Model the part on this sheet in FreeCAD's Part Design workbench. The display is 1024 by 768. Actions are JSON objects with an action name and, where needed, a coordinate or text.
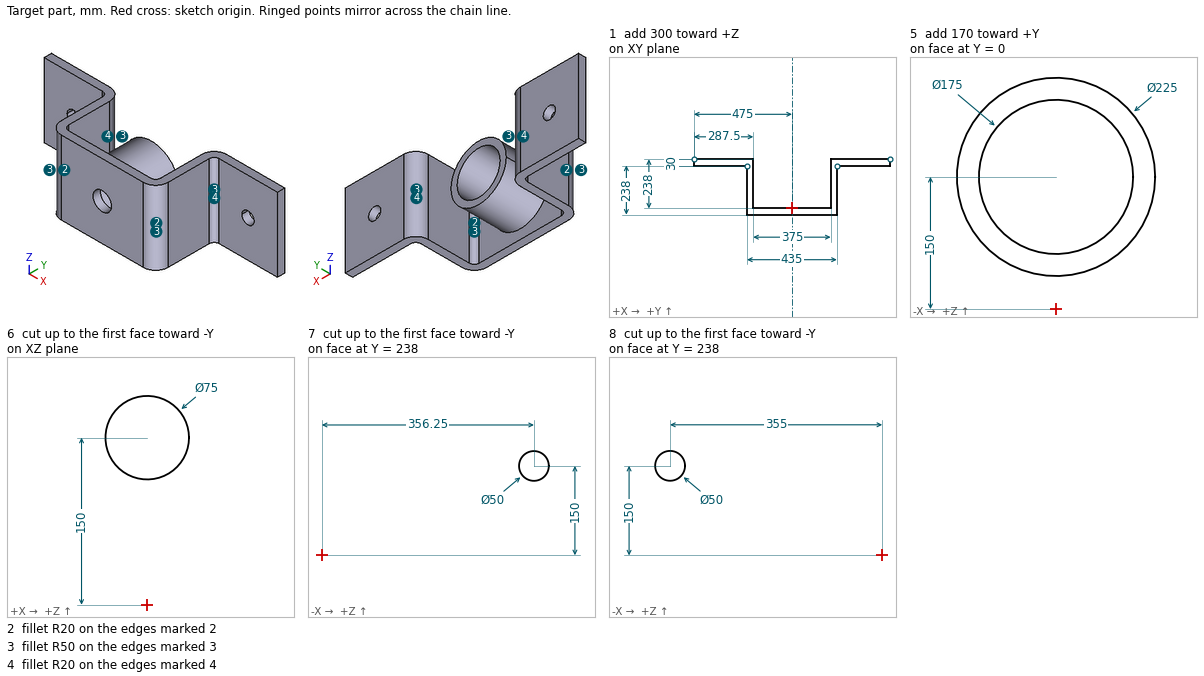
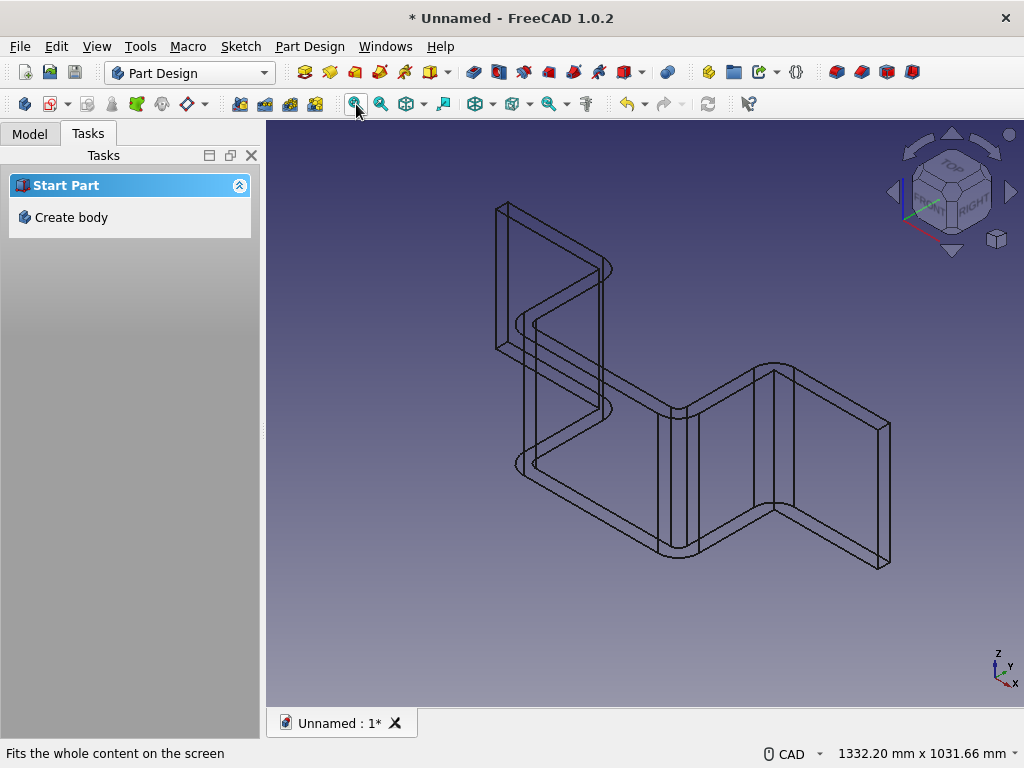
{"action": "left_click", "coordinate": [774, 439]}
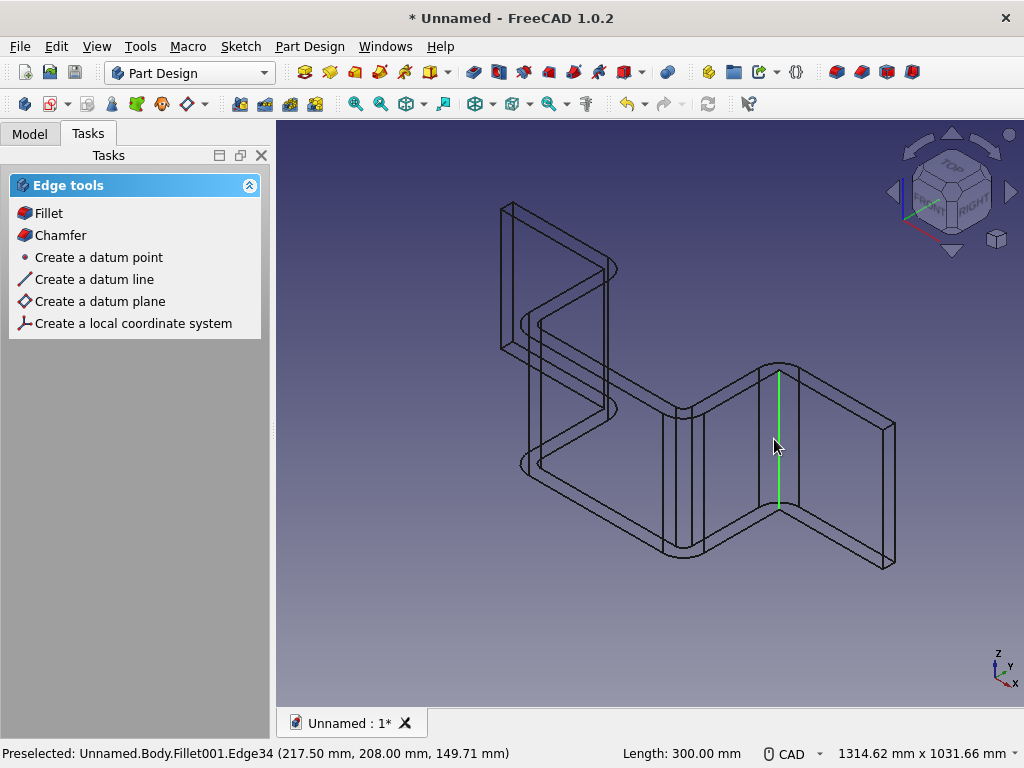
{"action": "scroll", "coordinate": [604, 338], "scroll_direction": "up", "scroll_amount": 6}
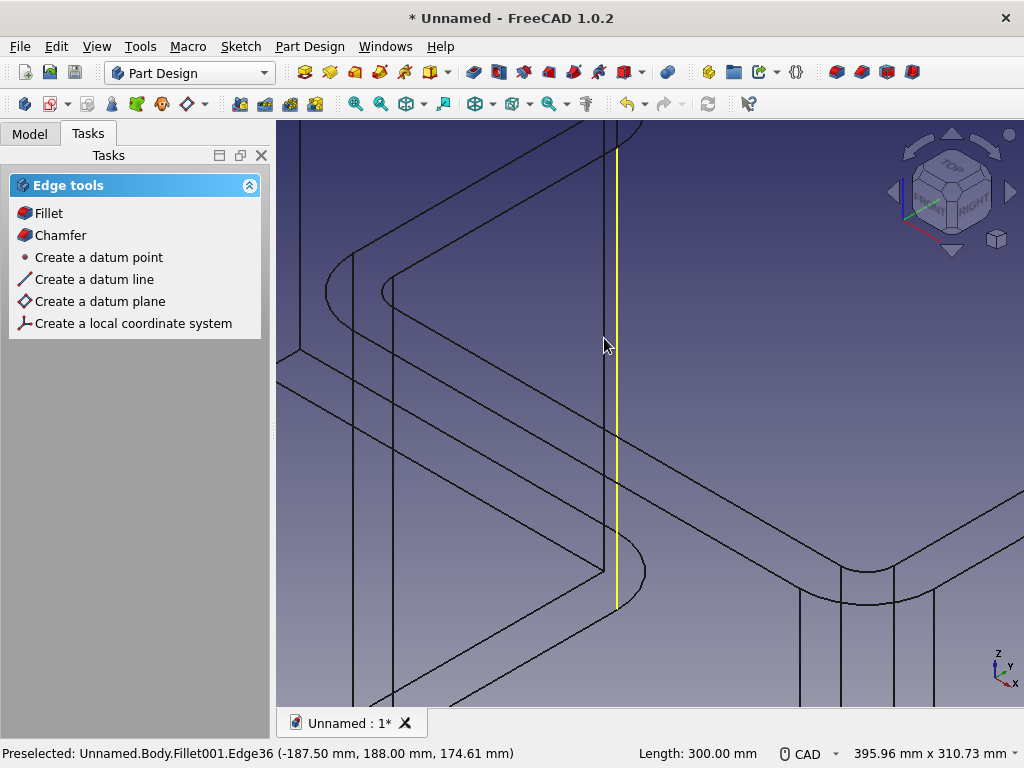
{"action": "left_click", "coordinate": [604, 339], "text": "ctrl"}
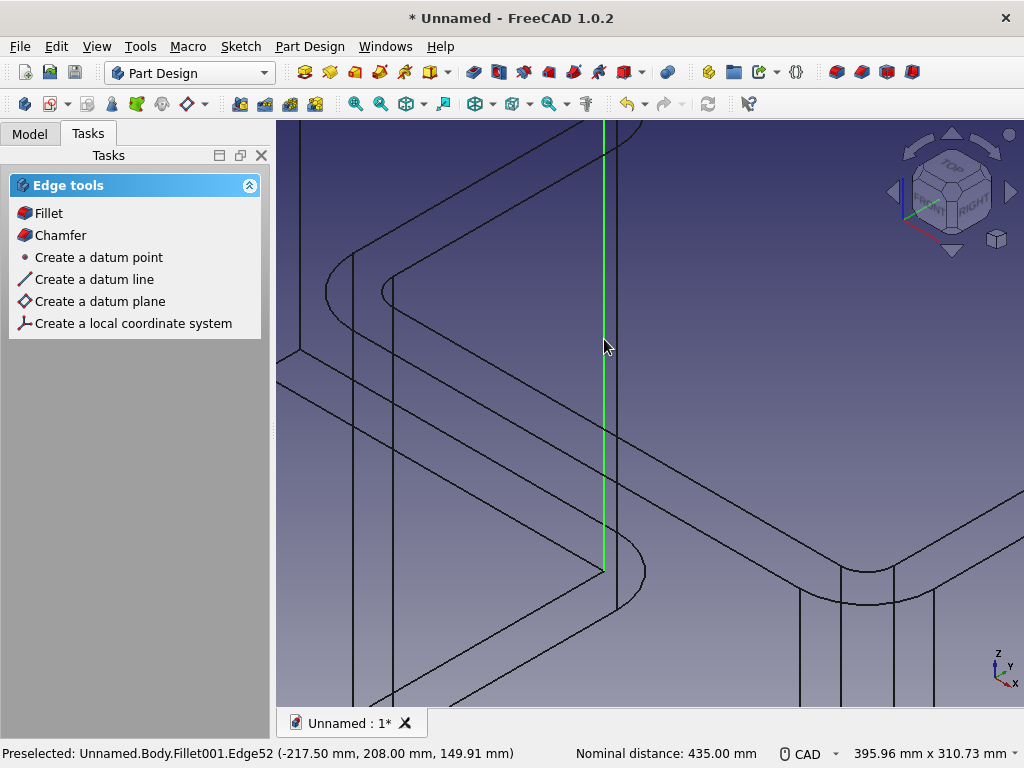
{"action": "key", "text": "v 1"}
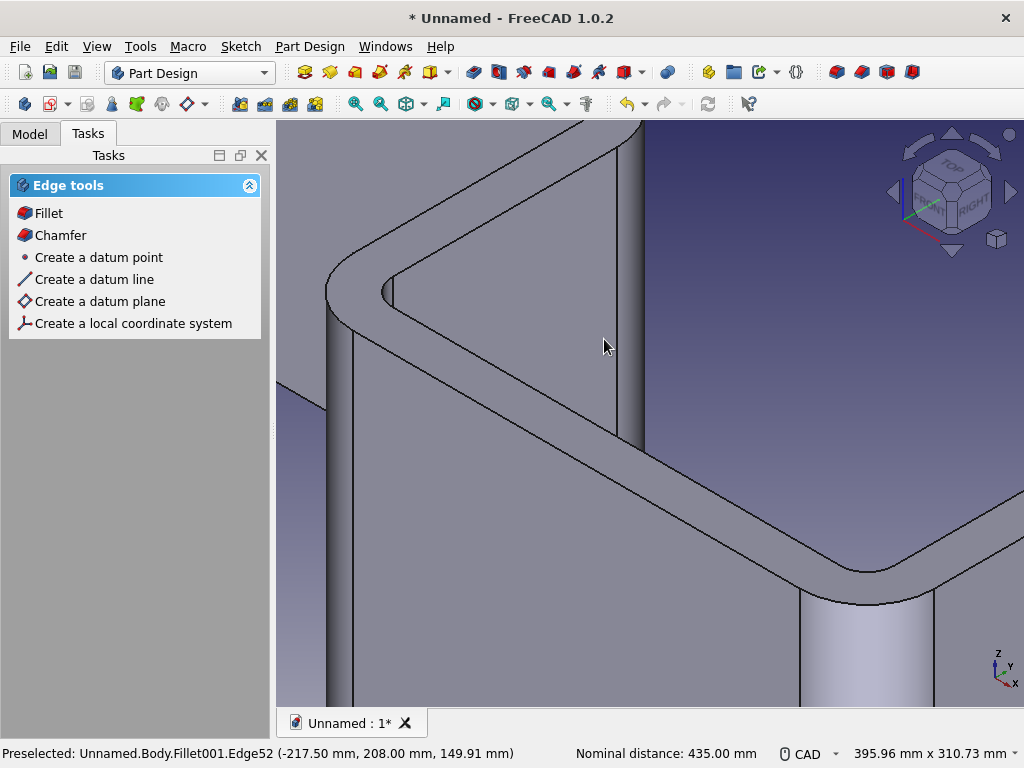
{"action": "left_click", "coordinate": [837, 72]}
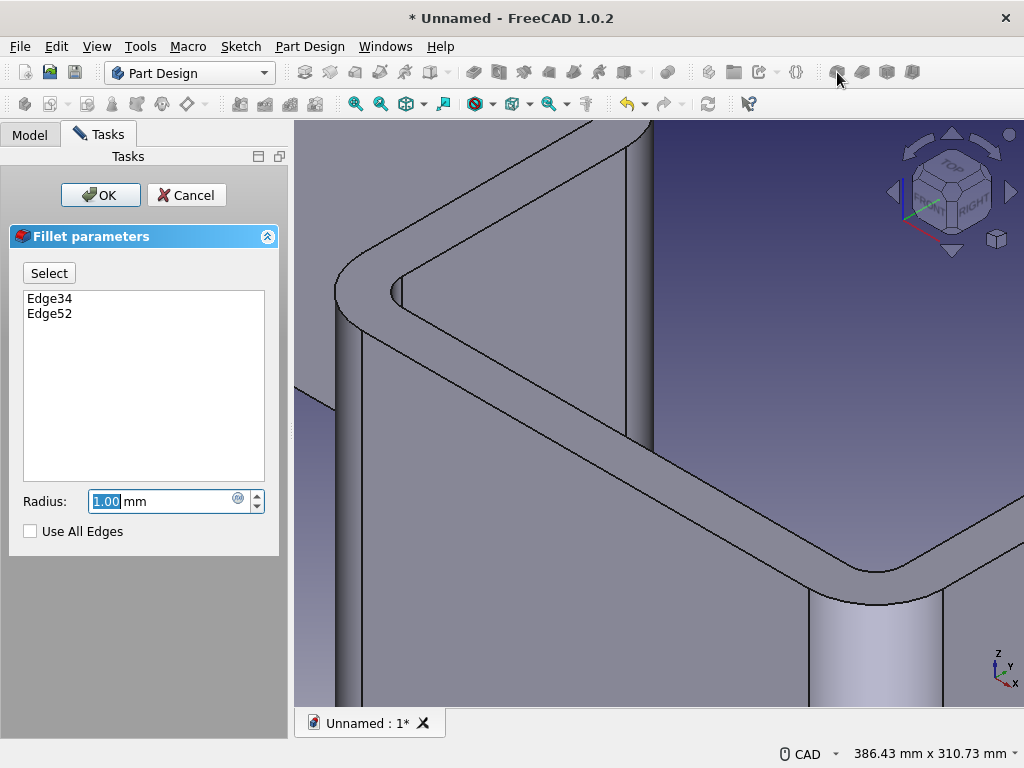
{"action": "type", "text": "20"}
{"action": "key", "text": "Tab"}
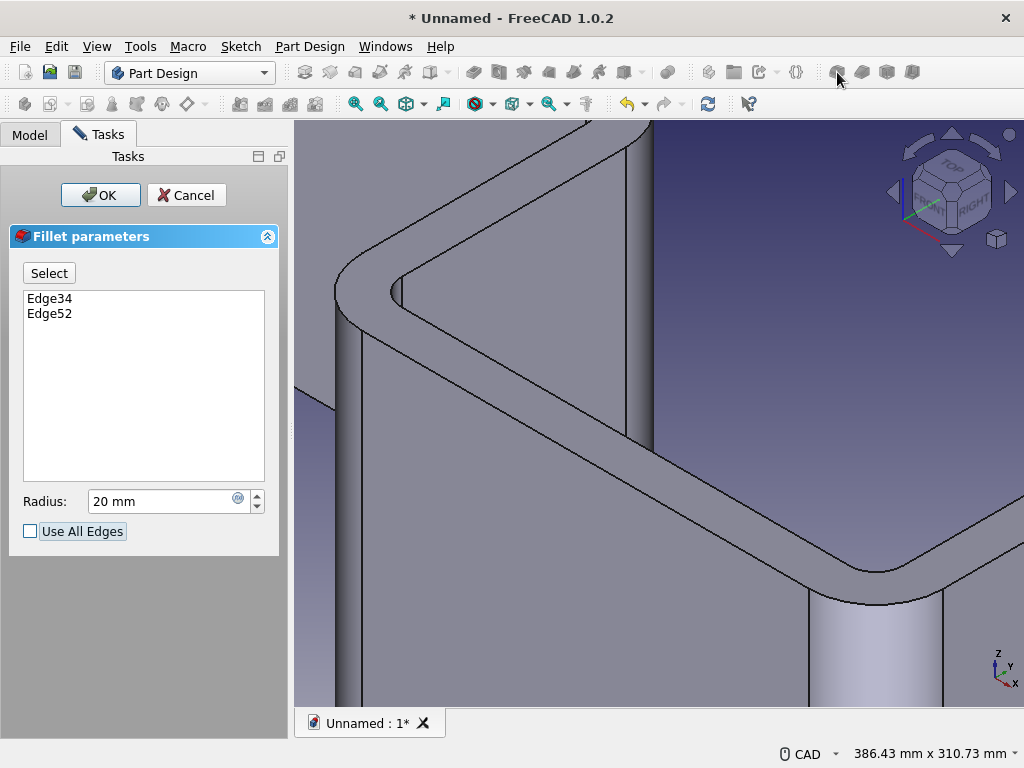
{"action": "left_click", "coordinate": [101, 195]}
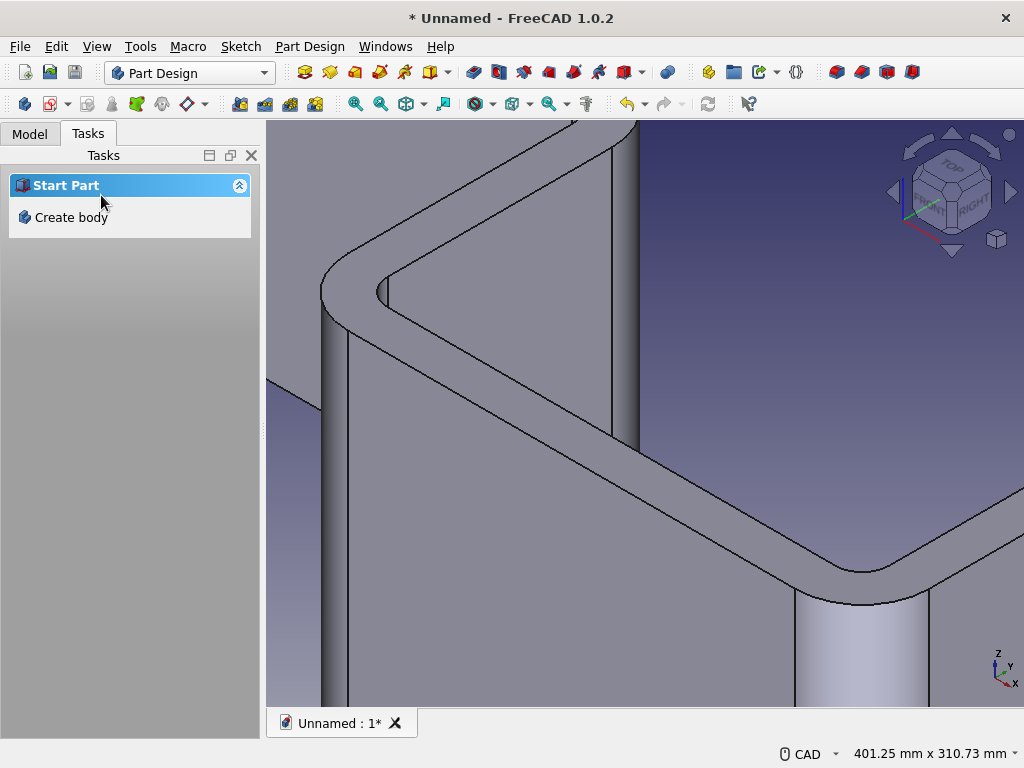
{"action": "left_click", "coordinate": [356, 104]}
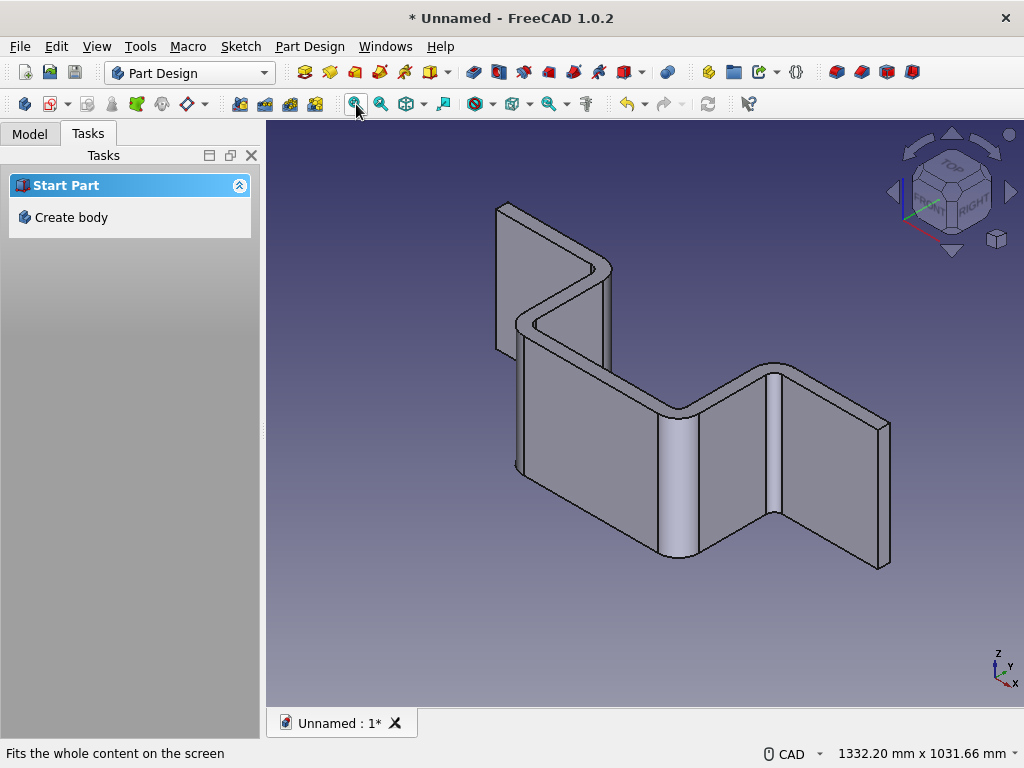
{"action": "key", "text": "4"}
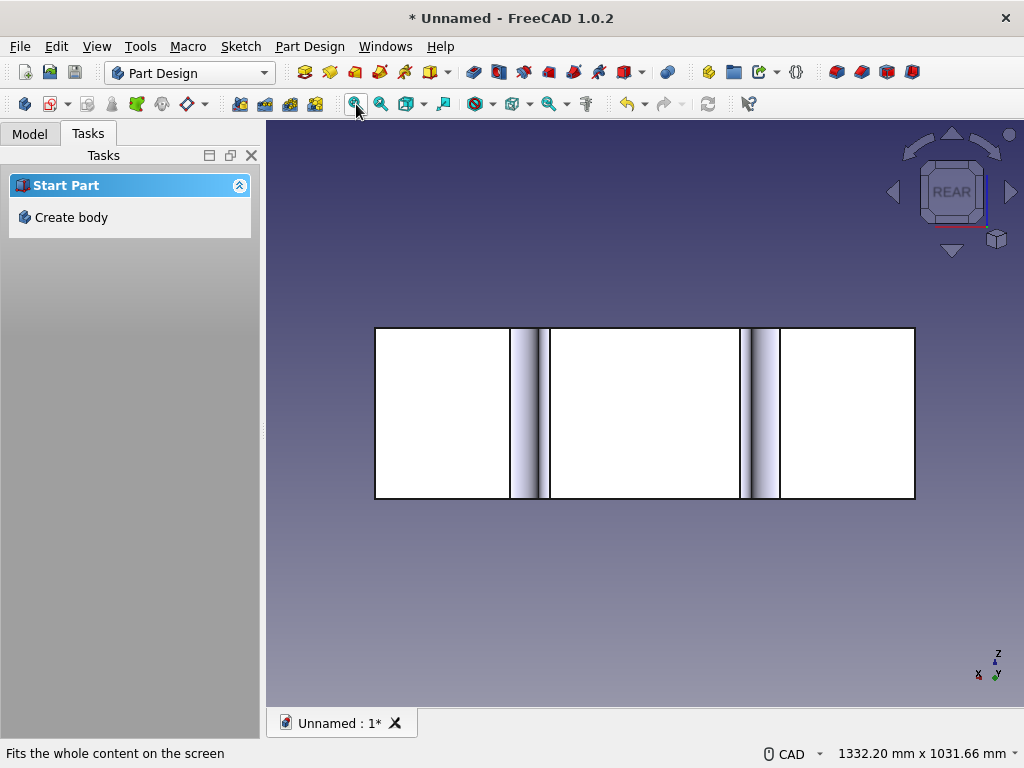
{"action": "left_click", "coordinate": [645, 412]}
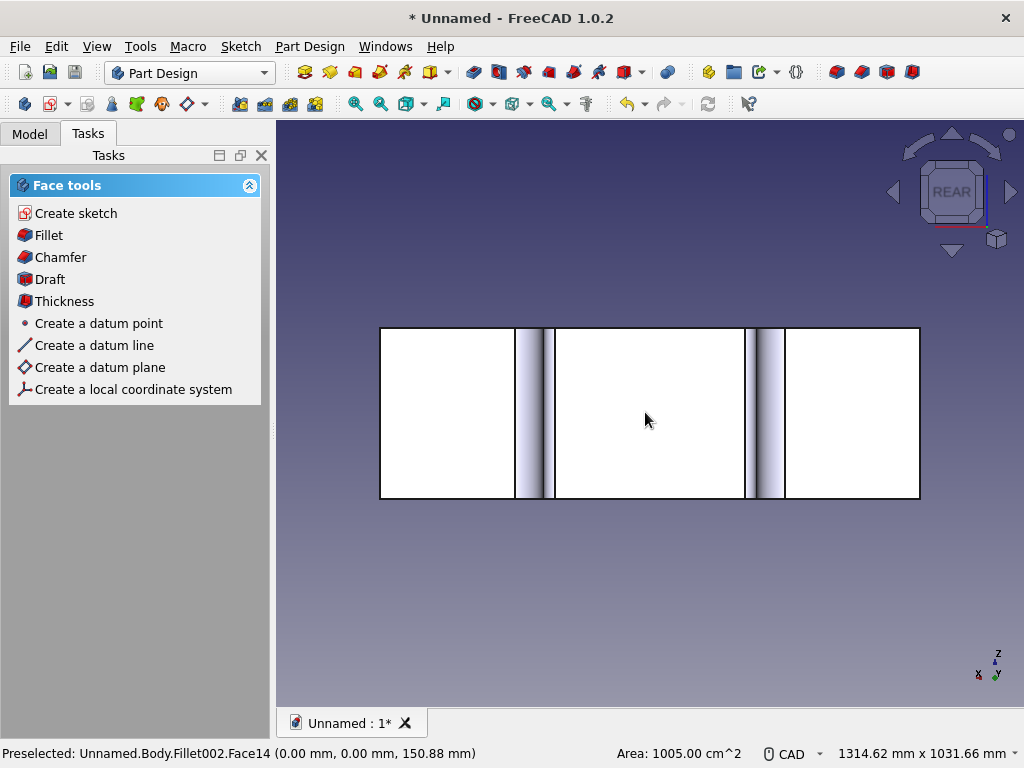
{"action": "left_click", "coordinate": [50, 104]}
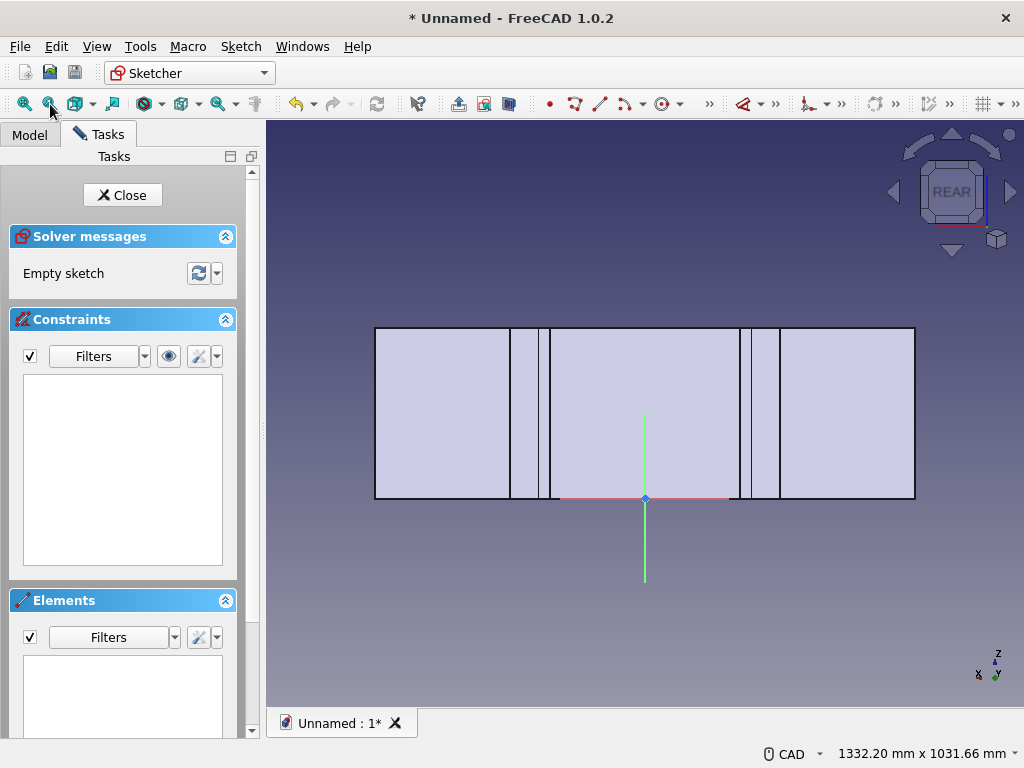
{"action": "left_click", "coordinate": [509, 104]}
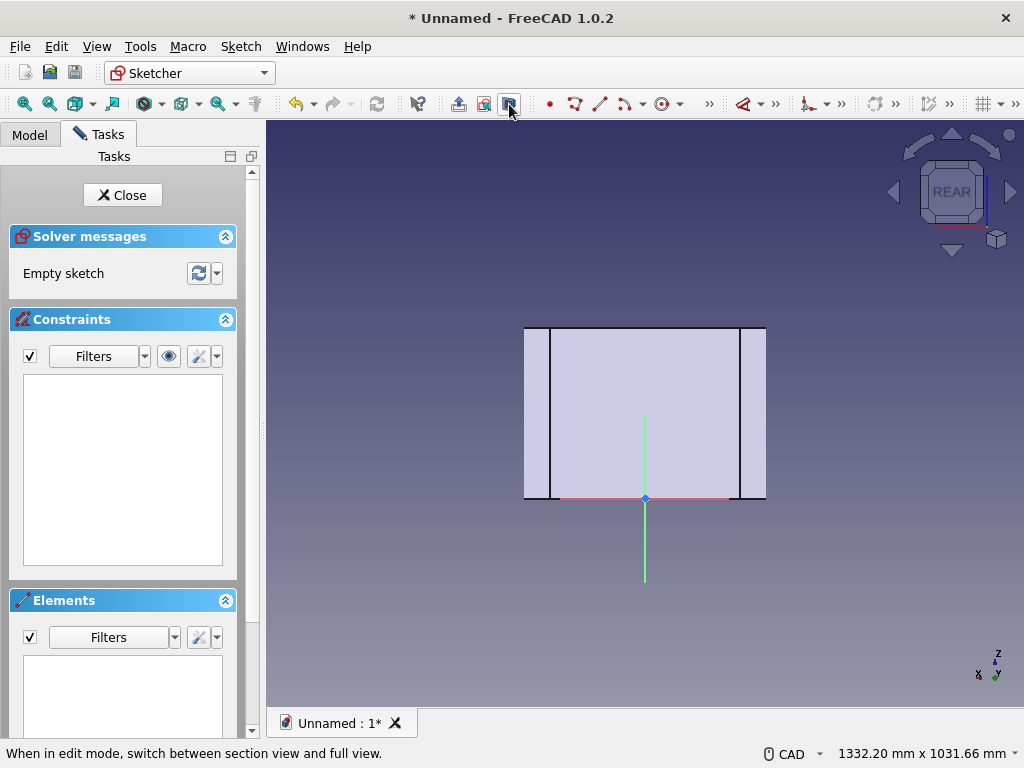
{"action": "scroll", "coordinate": [685, 430], "scroll_direction": "up", "scroll_amount": 5}